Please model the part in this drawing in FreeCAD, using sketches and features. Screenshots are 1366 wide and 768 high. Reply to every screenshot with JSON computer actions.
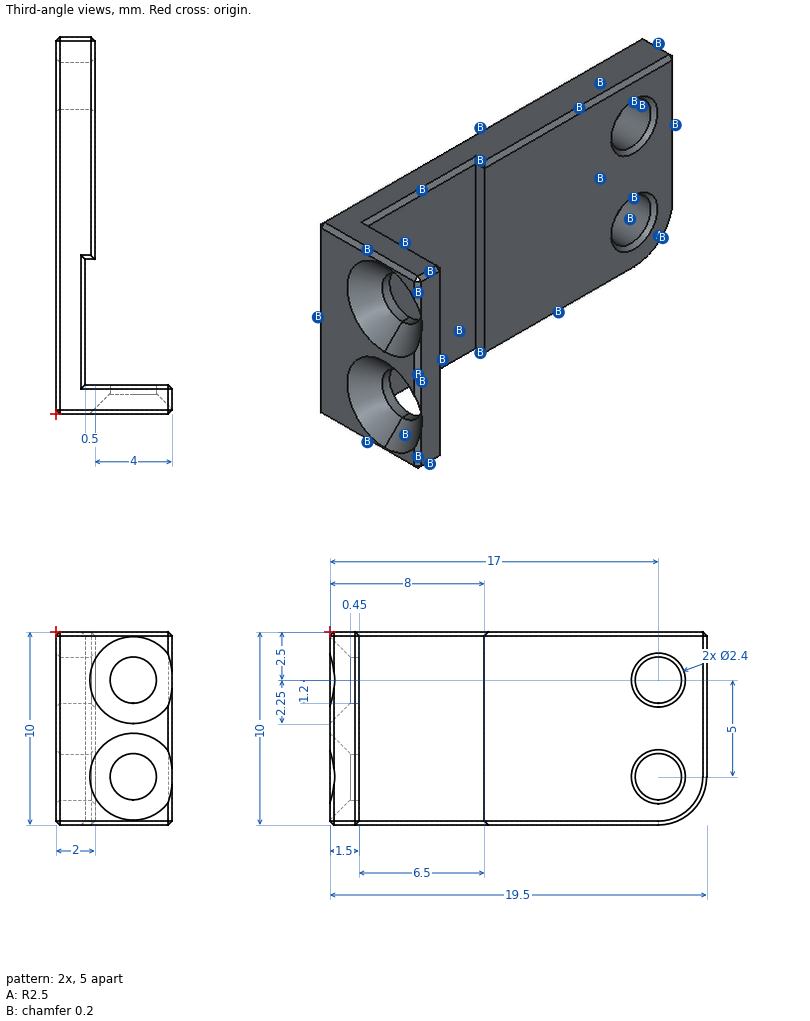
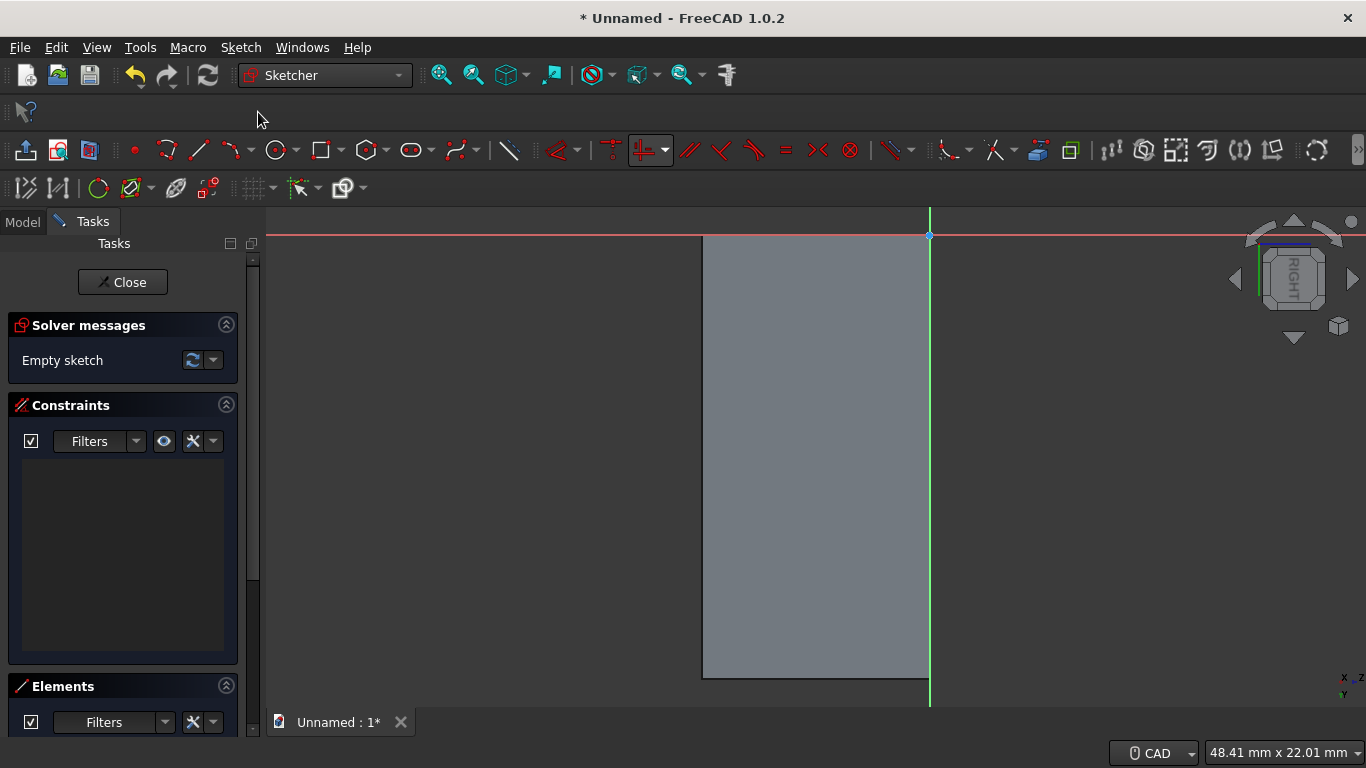
{"action": "scroll", "coordinate": [371, 524], "scroll_direction": "down", "scroll_amount": 1}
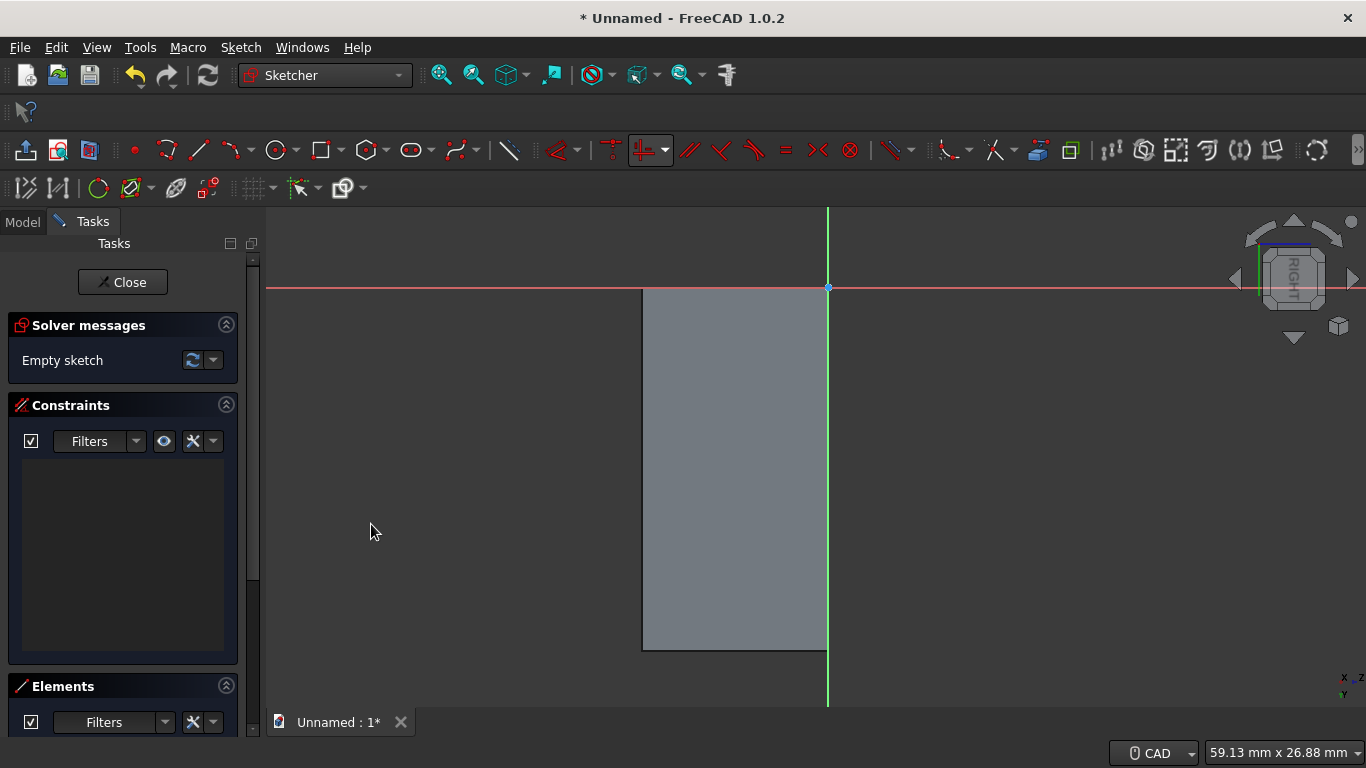
{"action": "left_click", "coordinate": [276, 150]}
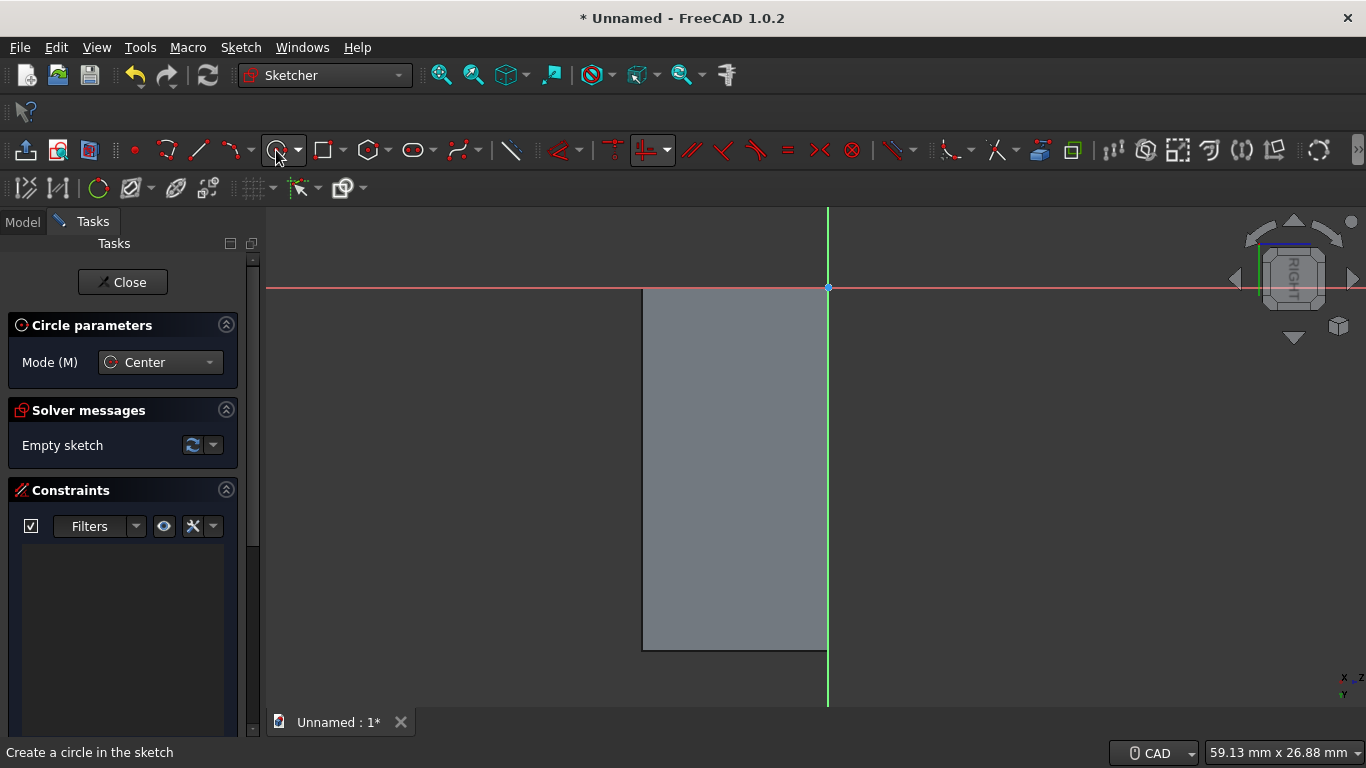
{"action": "left_click", "coordinate": [782, 604]}
{"action": "left_click", "coordinate": [798, 588]}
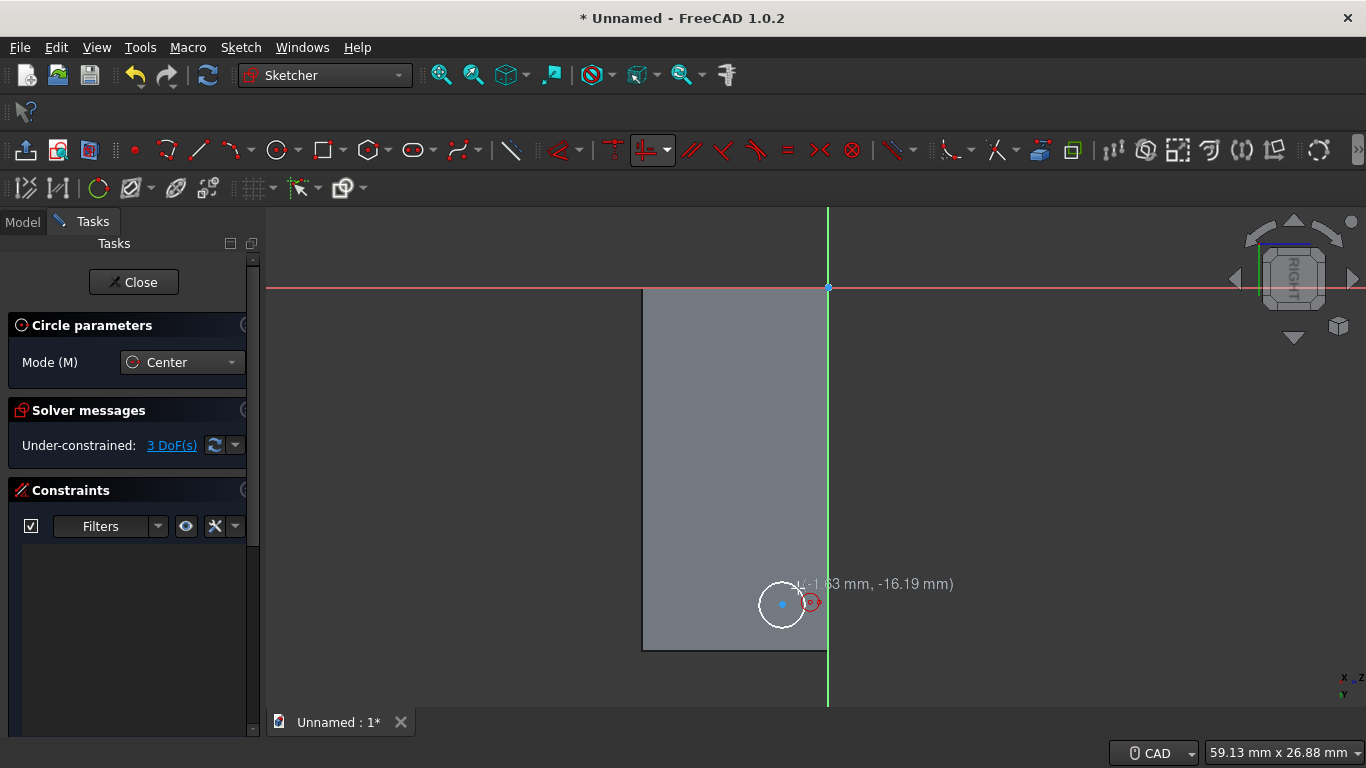
{"action": "left_click", "coordinate": [689, 604]}
{"action": "left_click", "coordinate": [705, 588]}
{"action": "key", "text": "Escape"}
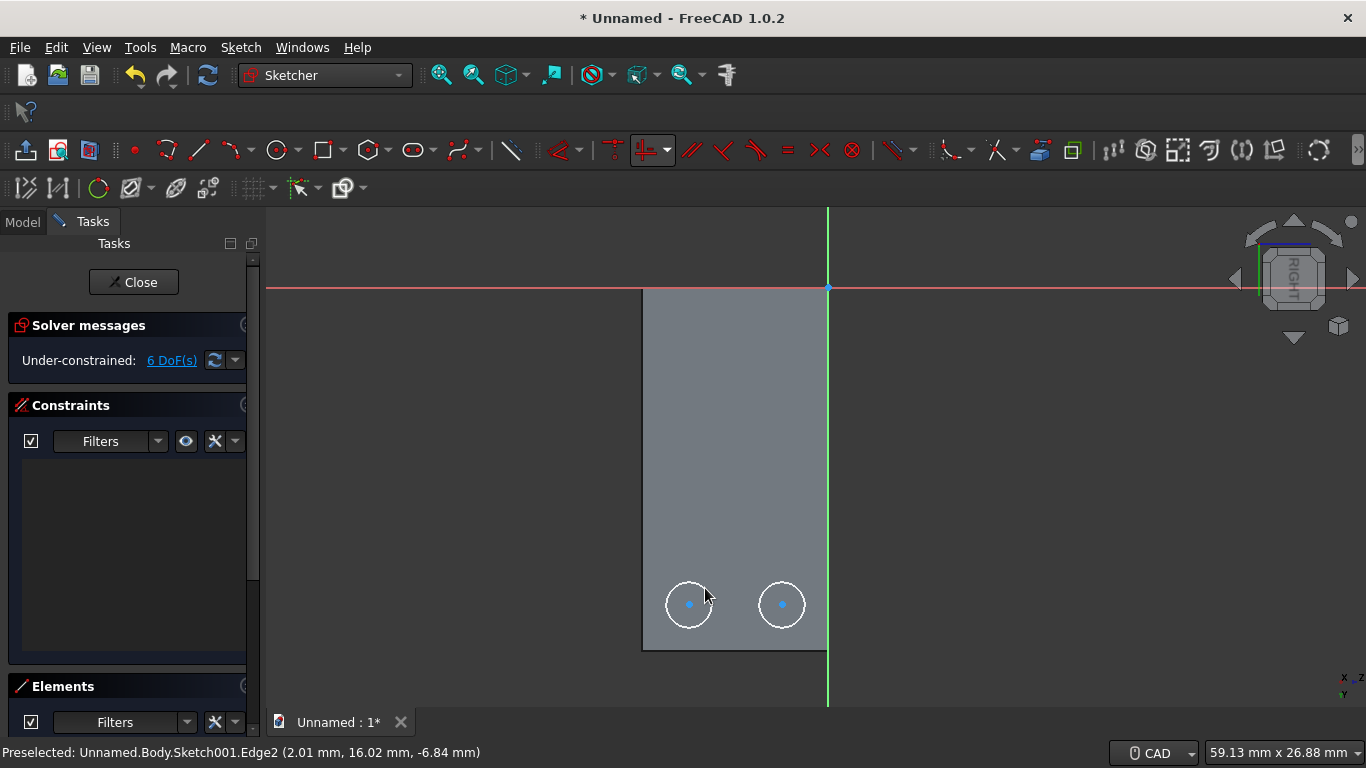
{"action": "left_click", "coordinate": [798, 589]}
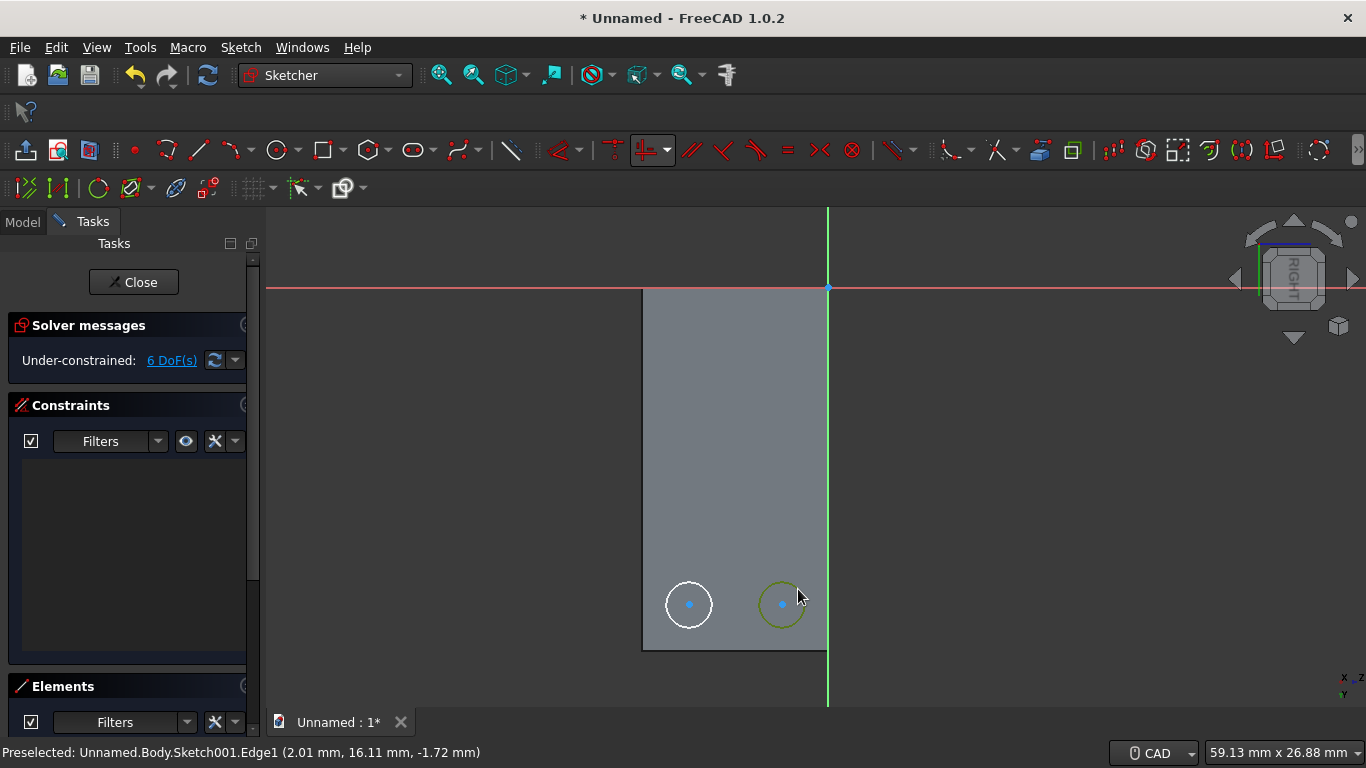
{"action": "left_click", "coordinate": [705, 589]}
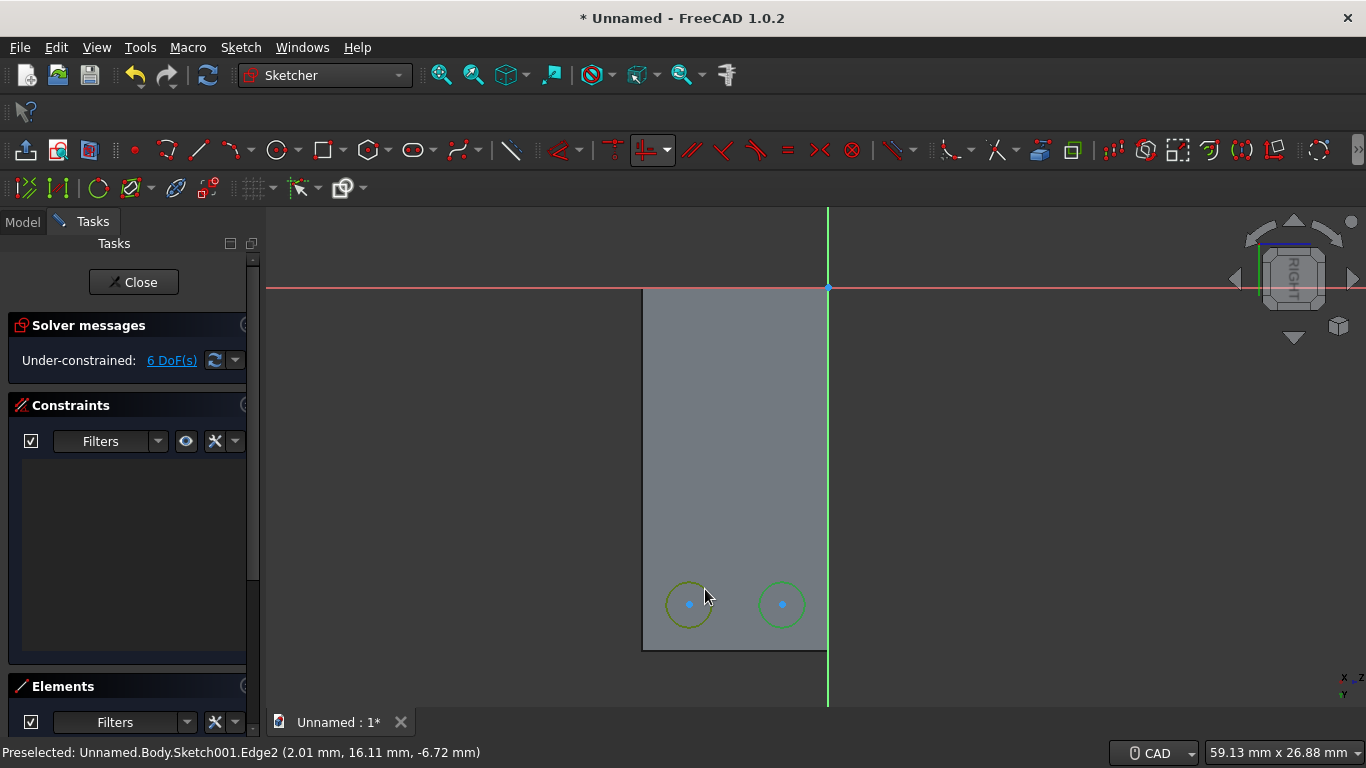
{"action": "left_click", "coordinate": [788, 150]}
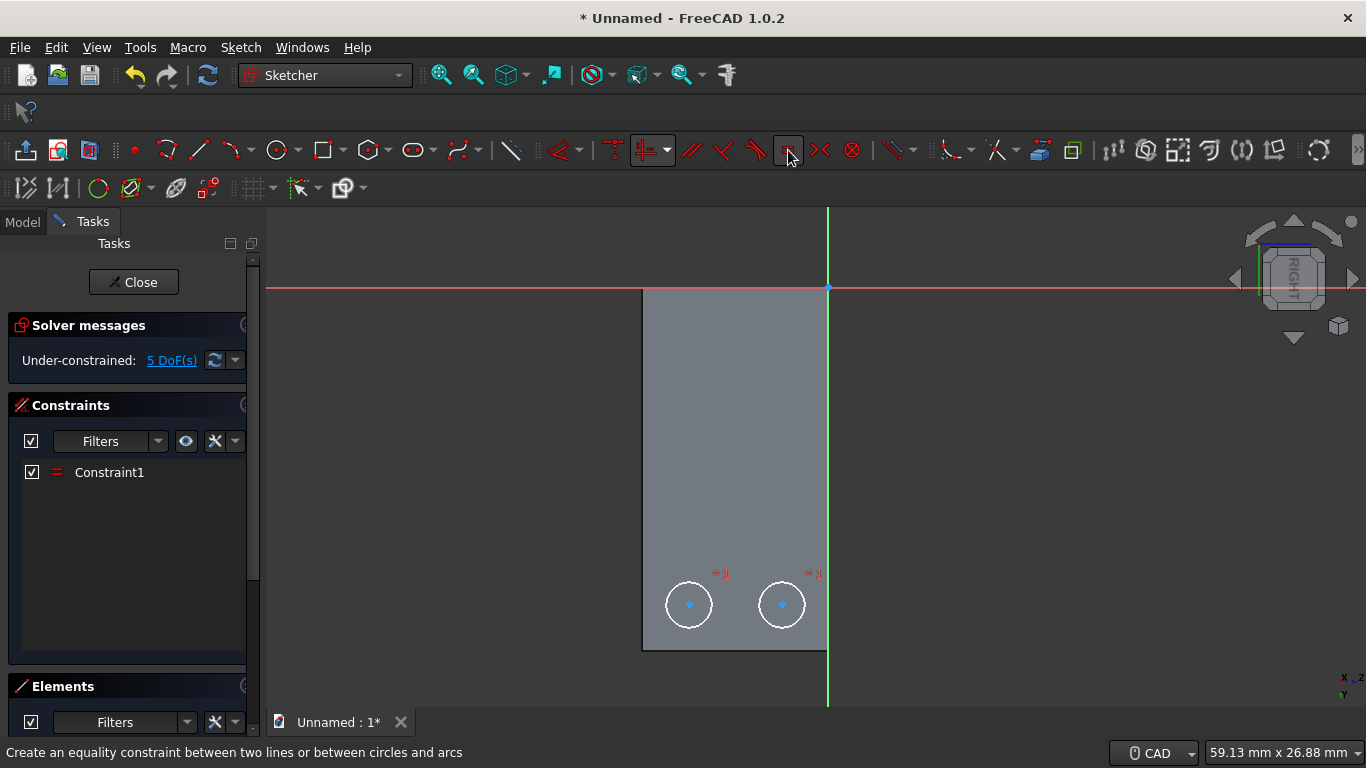
{"action": "left_click", "coordinate": [782, 605]}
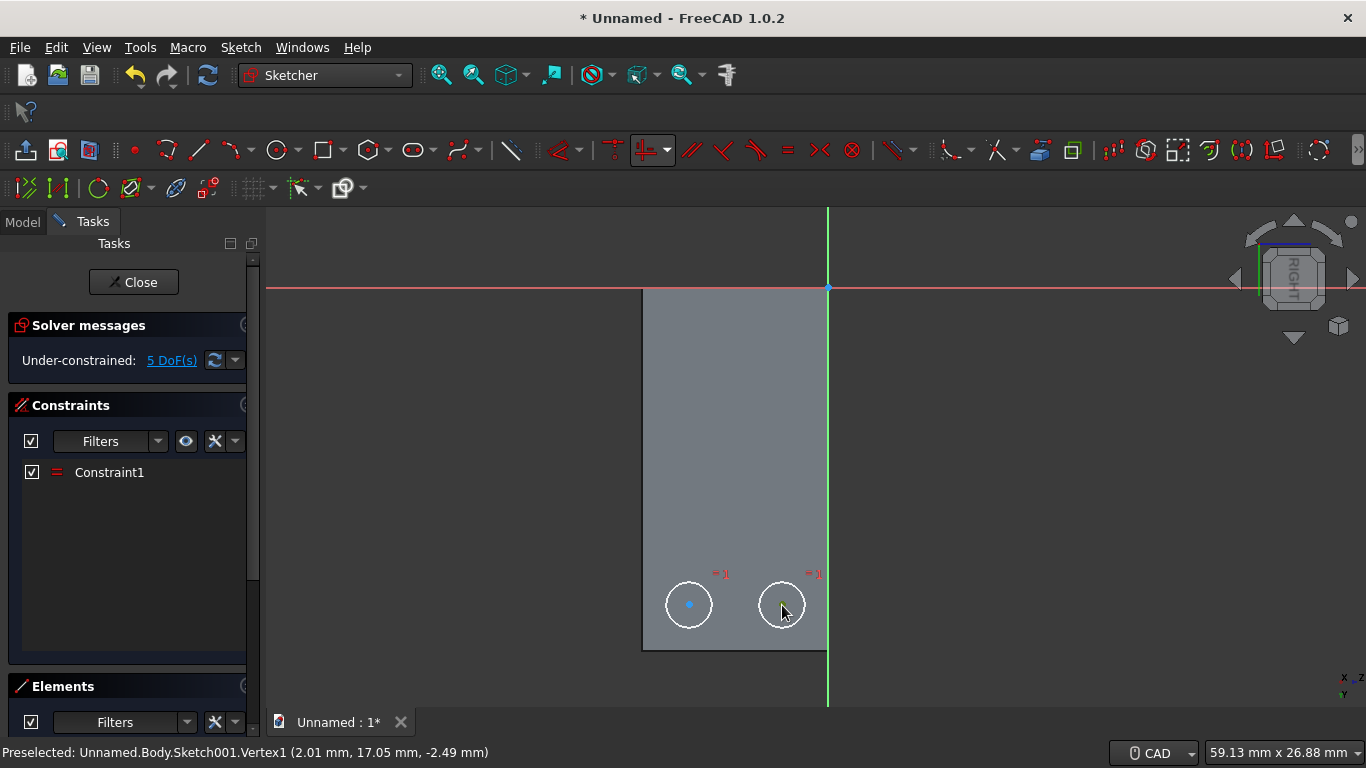
{"action": "left_click", "coordinate": [689, 605]}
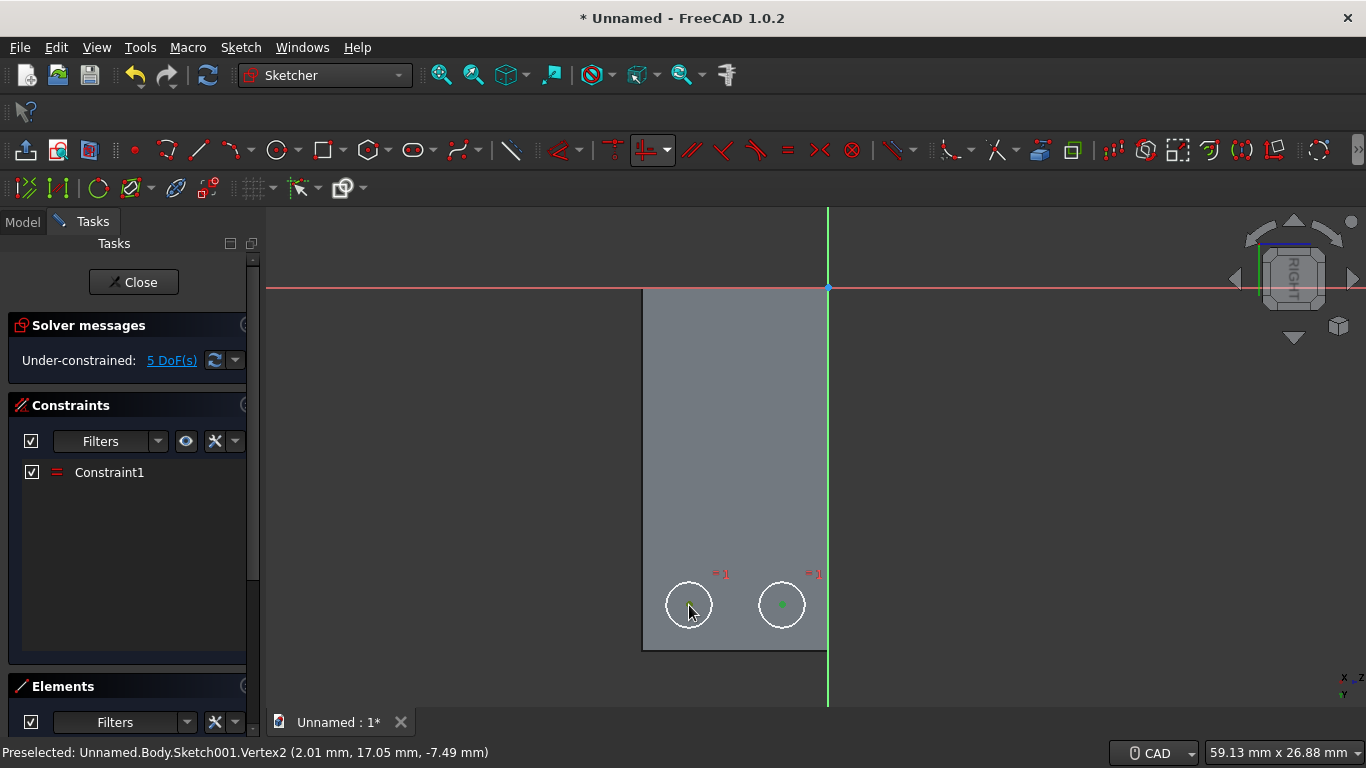
{"action": "key", "text": "h"}